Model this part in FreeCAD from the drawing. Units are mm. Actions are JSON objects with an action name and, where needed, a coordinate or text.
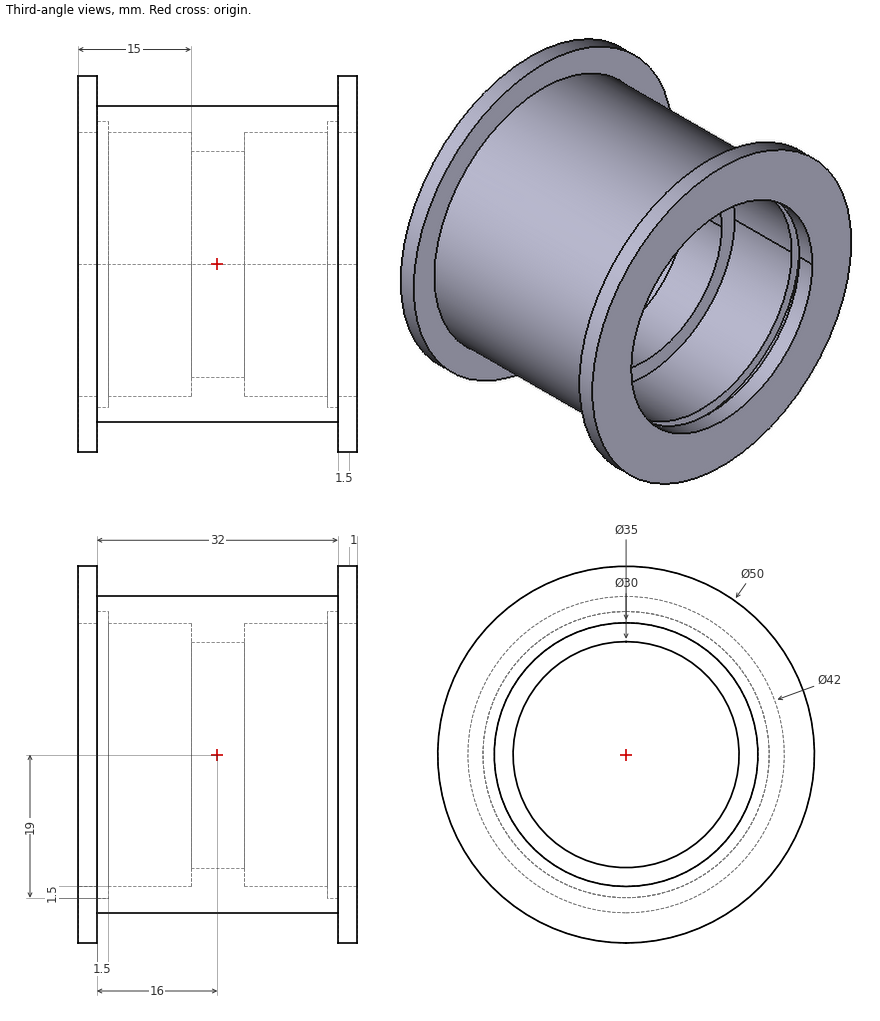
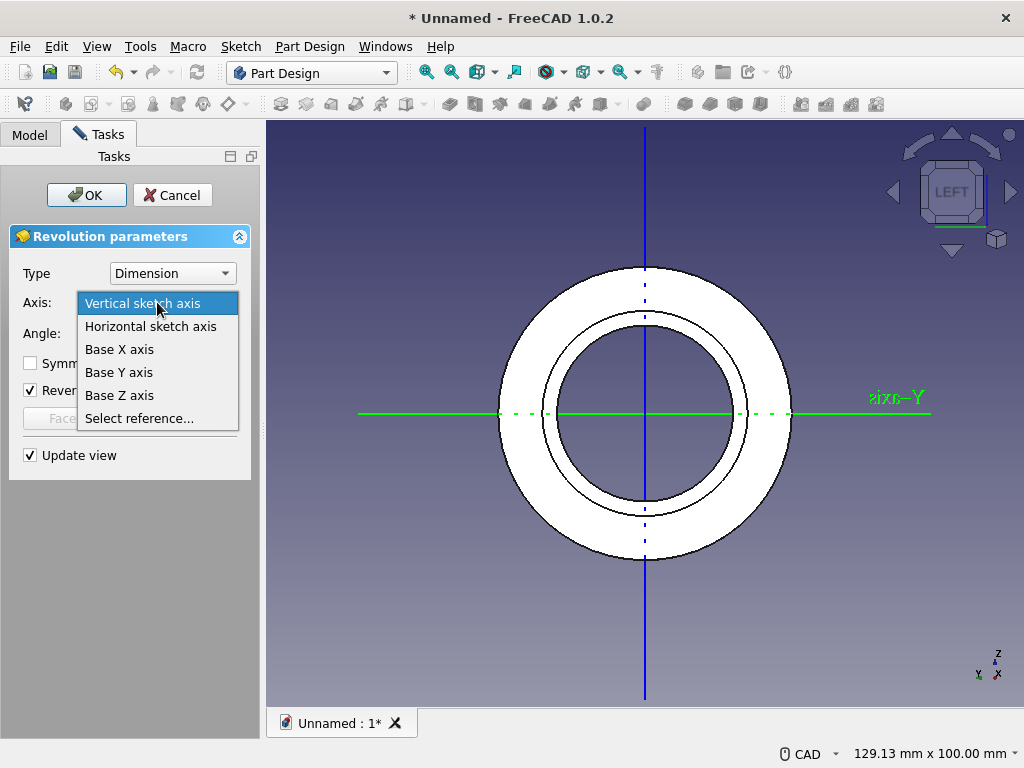
{"action": "left_click", "coordinate": [156, 326]}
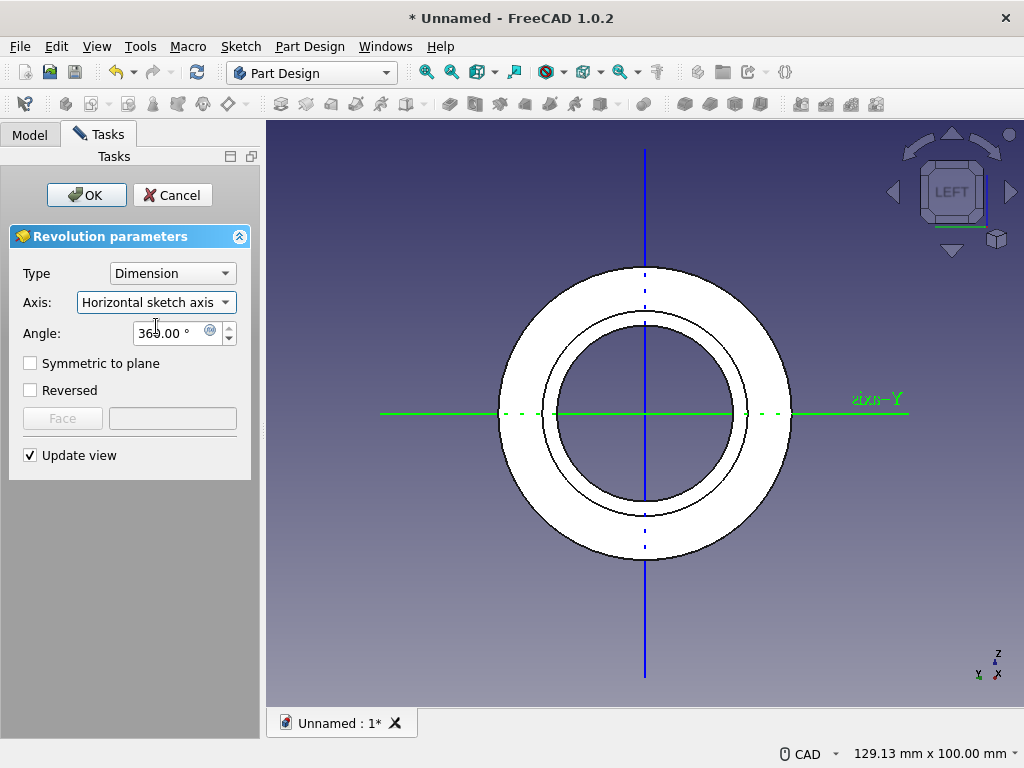
{"action": "left_click", "coordinate": [87, 195]}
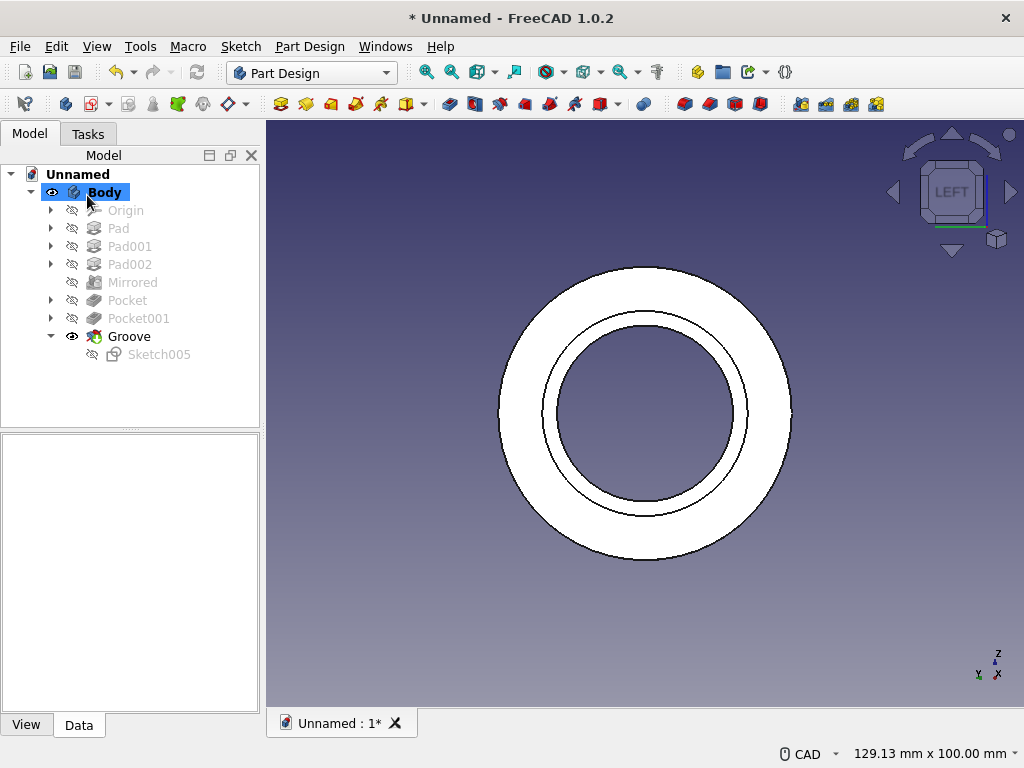
{"action": "left_click", "coordinate": [117, 318]}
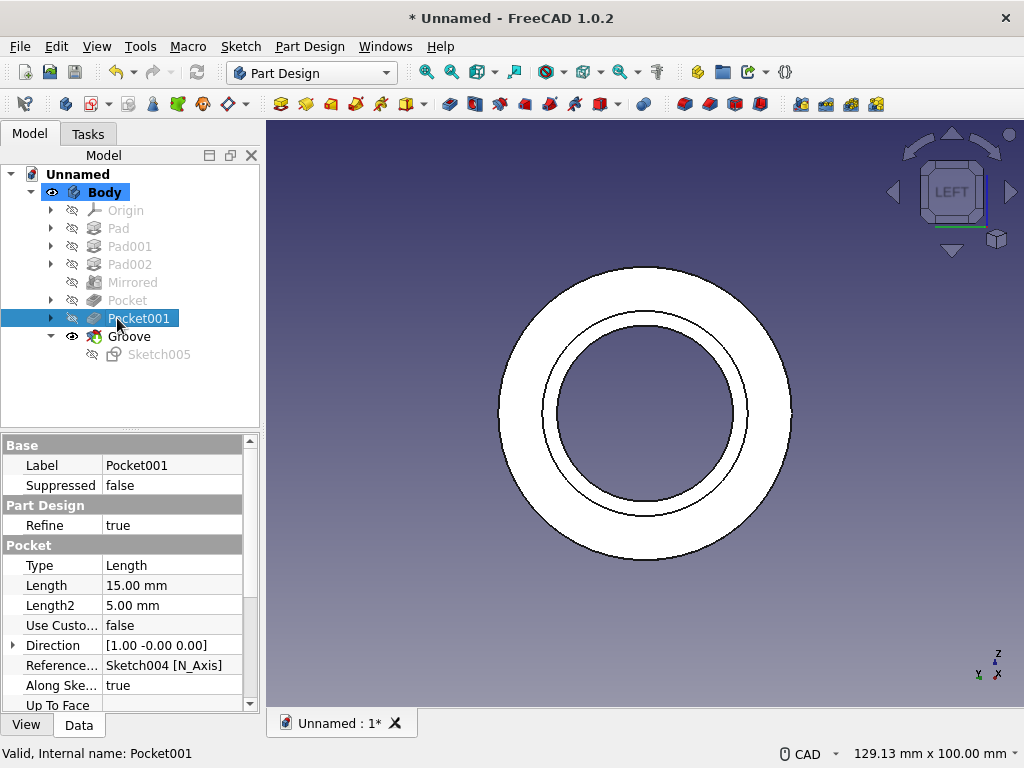
{"action": "left_click", "coordinate": [117, 336], "text": "ctrl"}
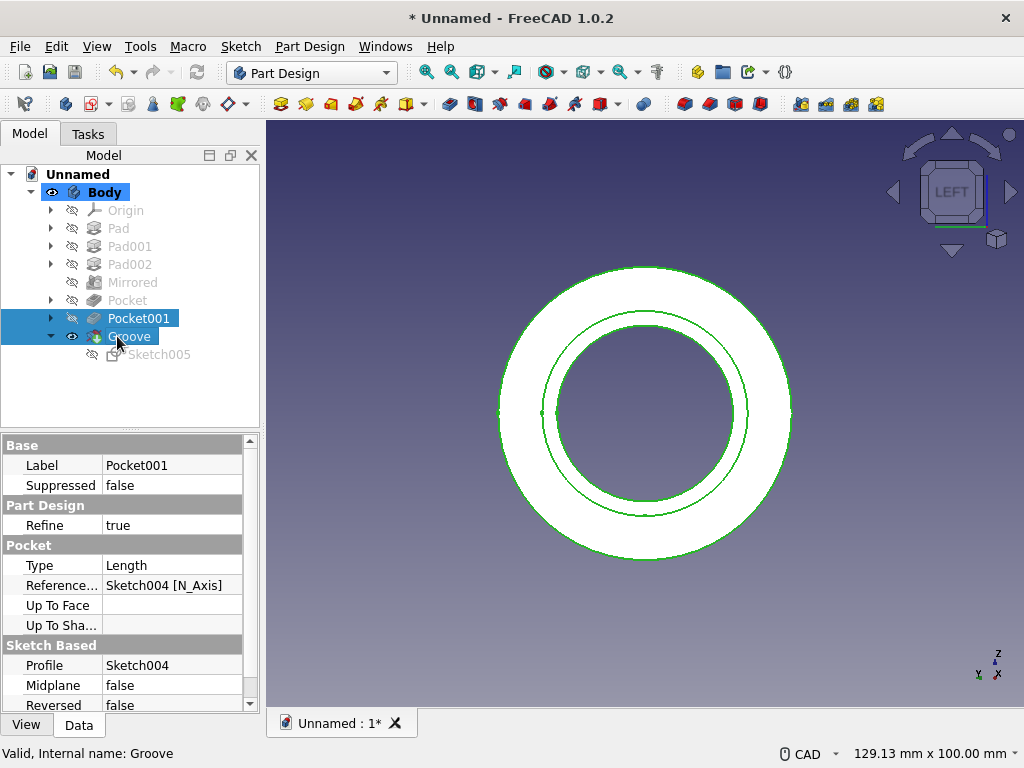
{"action": "left_click", "coordinate": [801, 104]}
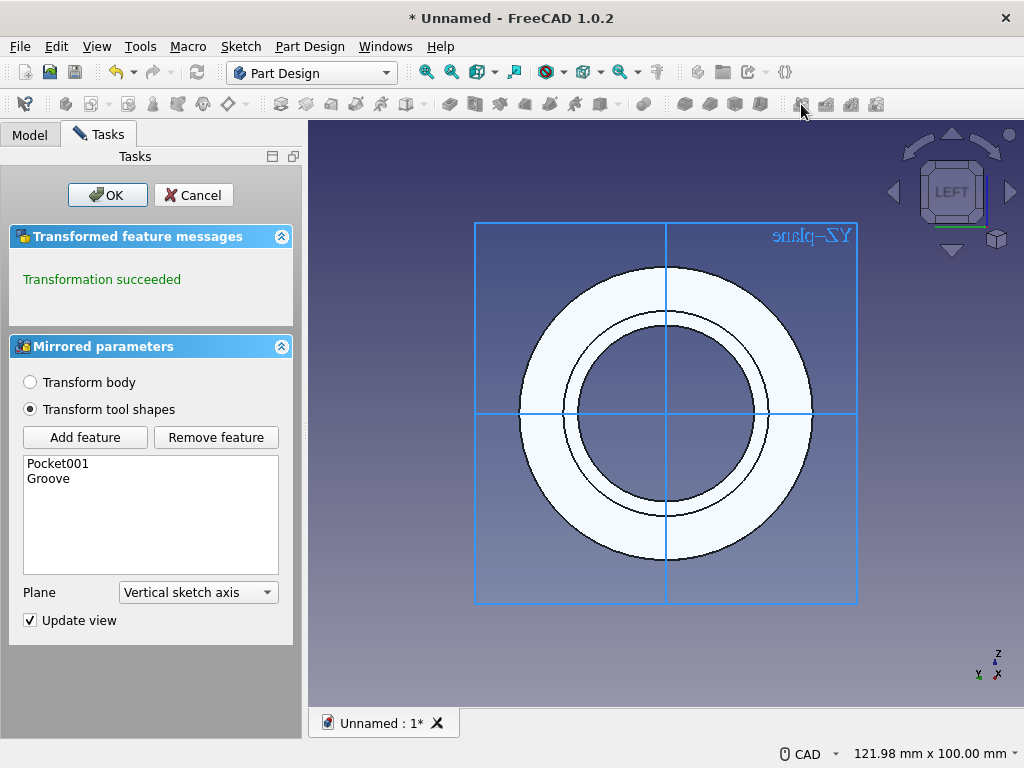
{"action": "left_click", "coordinate": [199, 592]}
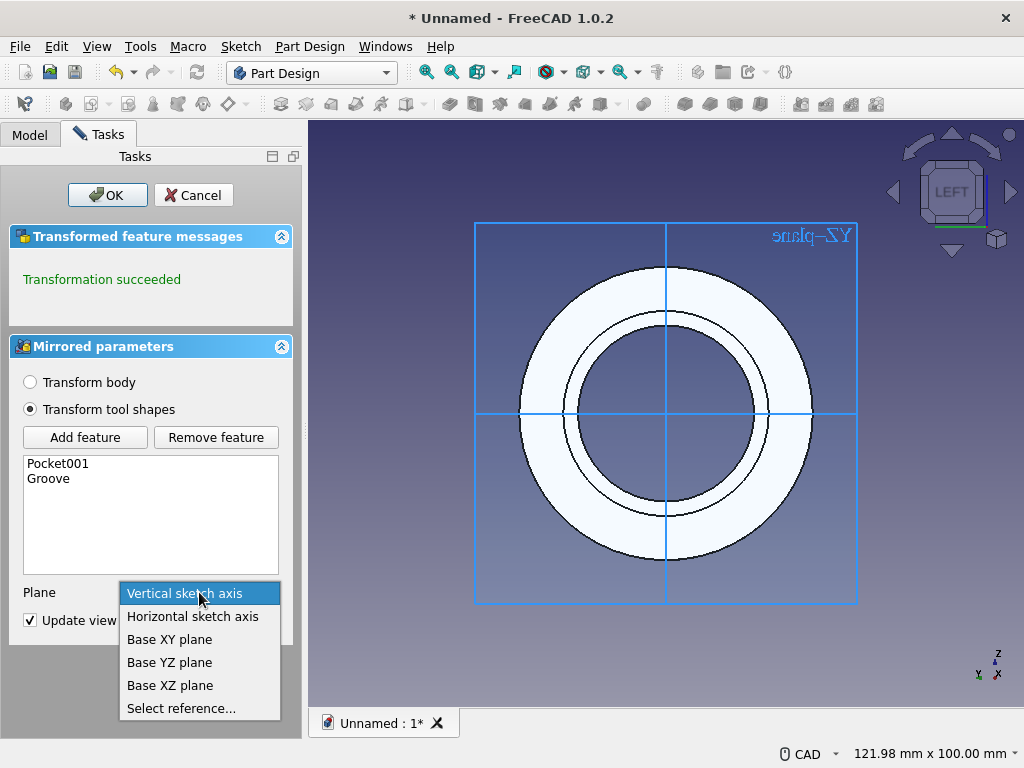
{"action": "left_click", "coordinate": [198, 662]}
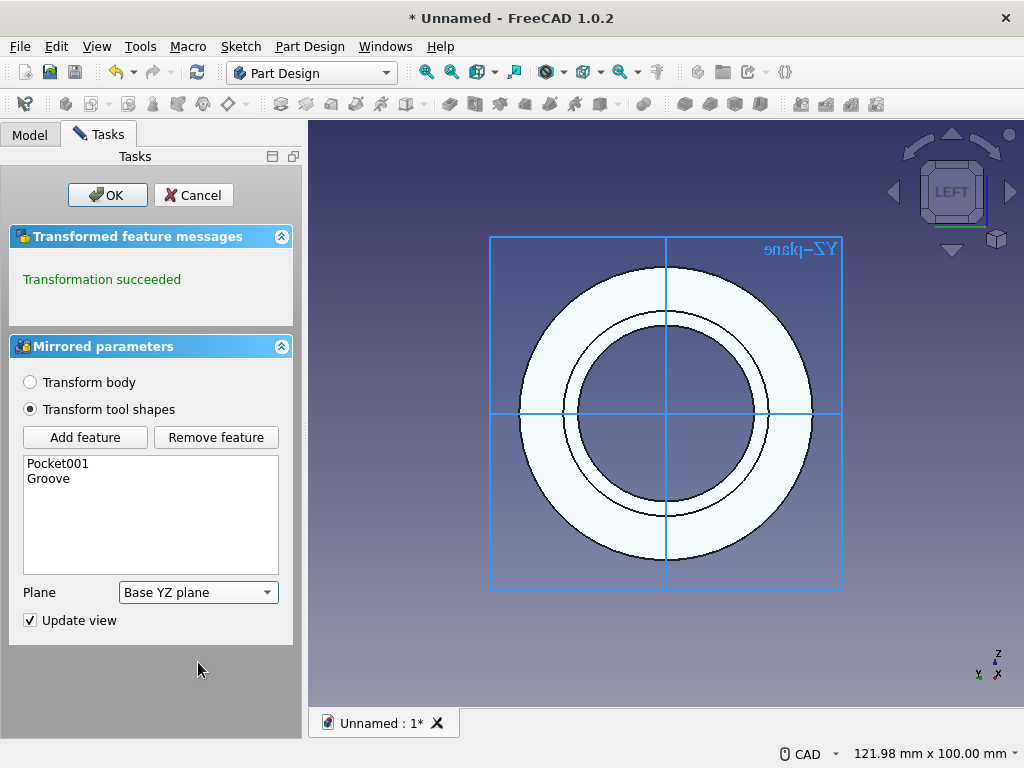
{"action": "left_click", "coordinate": [108, 195]}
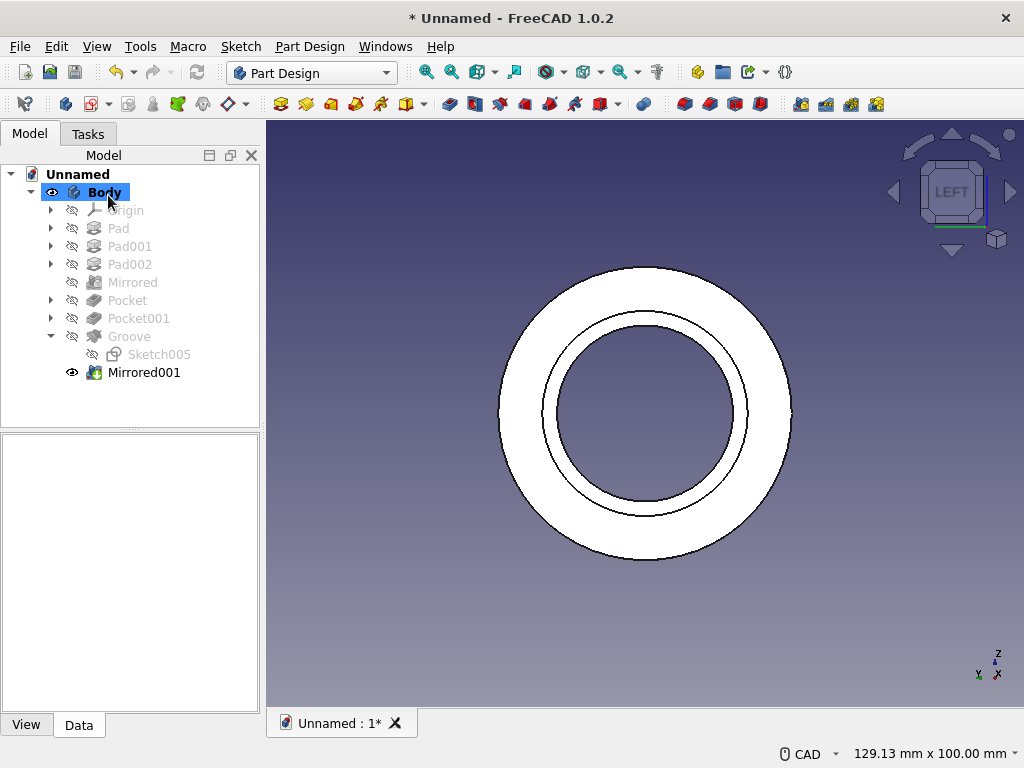
{"action": "key", "text": "0"}